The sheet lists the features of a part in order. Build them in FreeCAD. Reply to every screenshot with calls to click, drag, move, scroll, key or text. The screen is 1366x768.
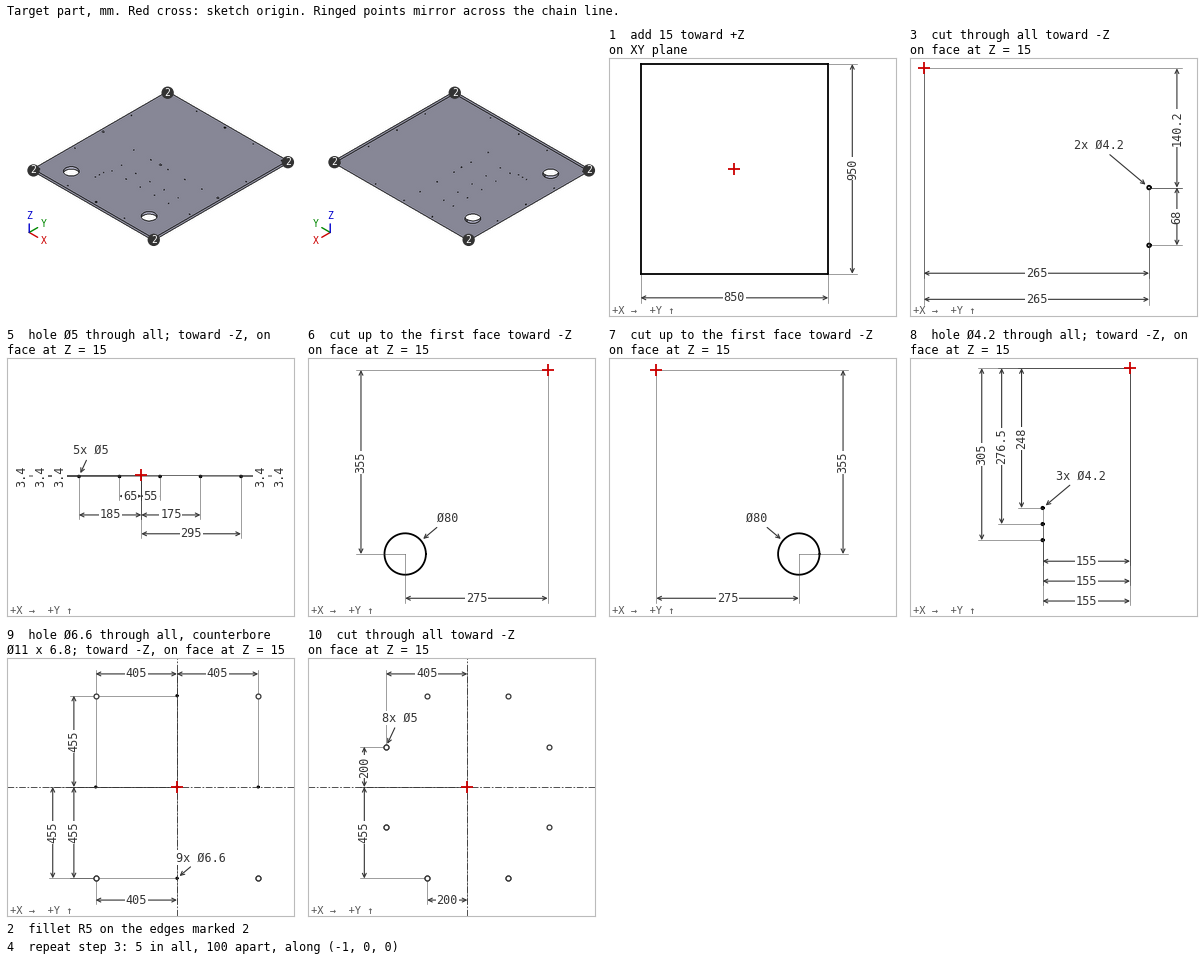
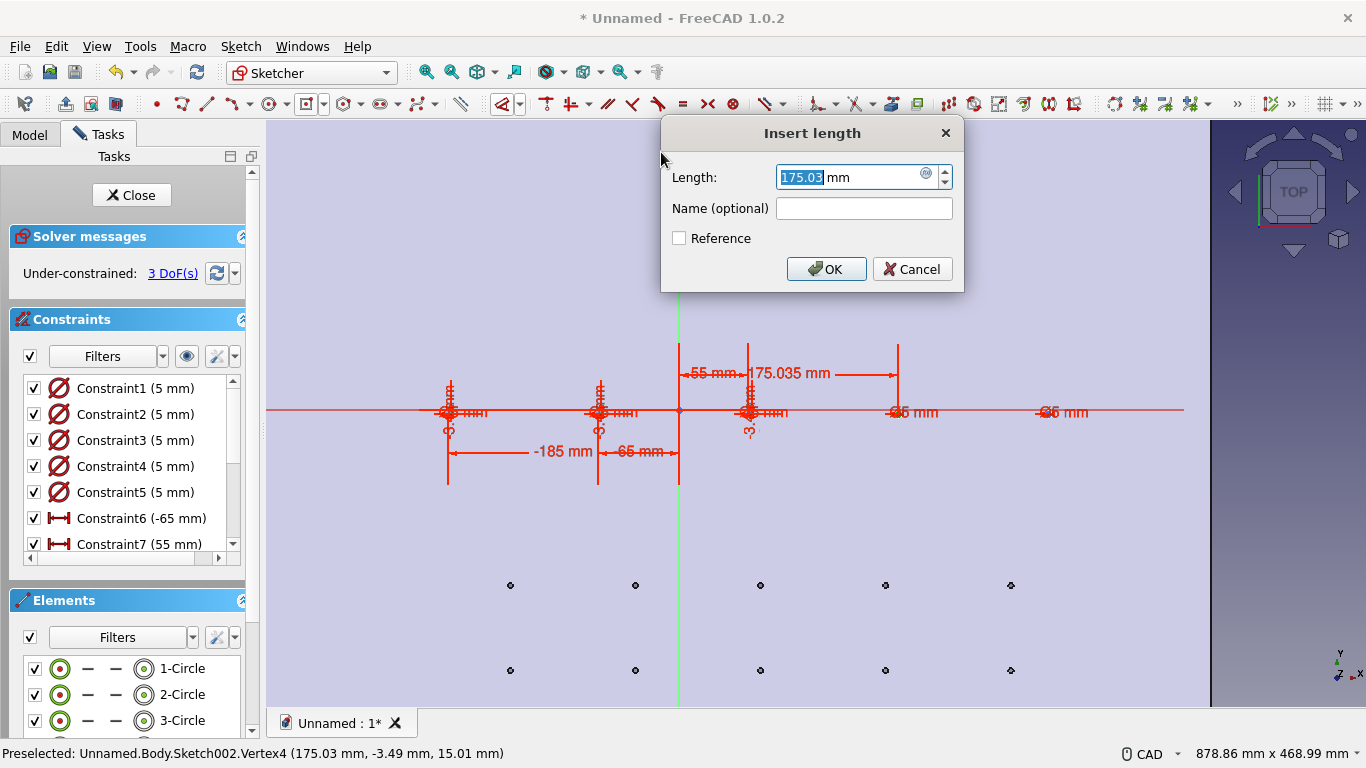
text(175)
key(Return)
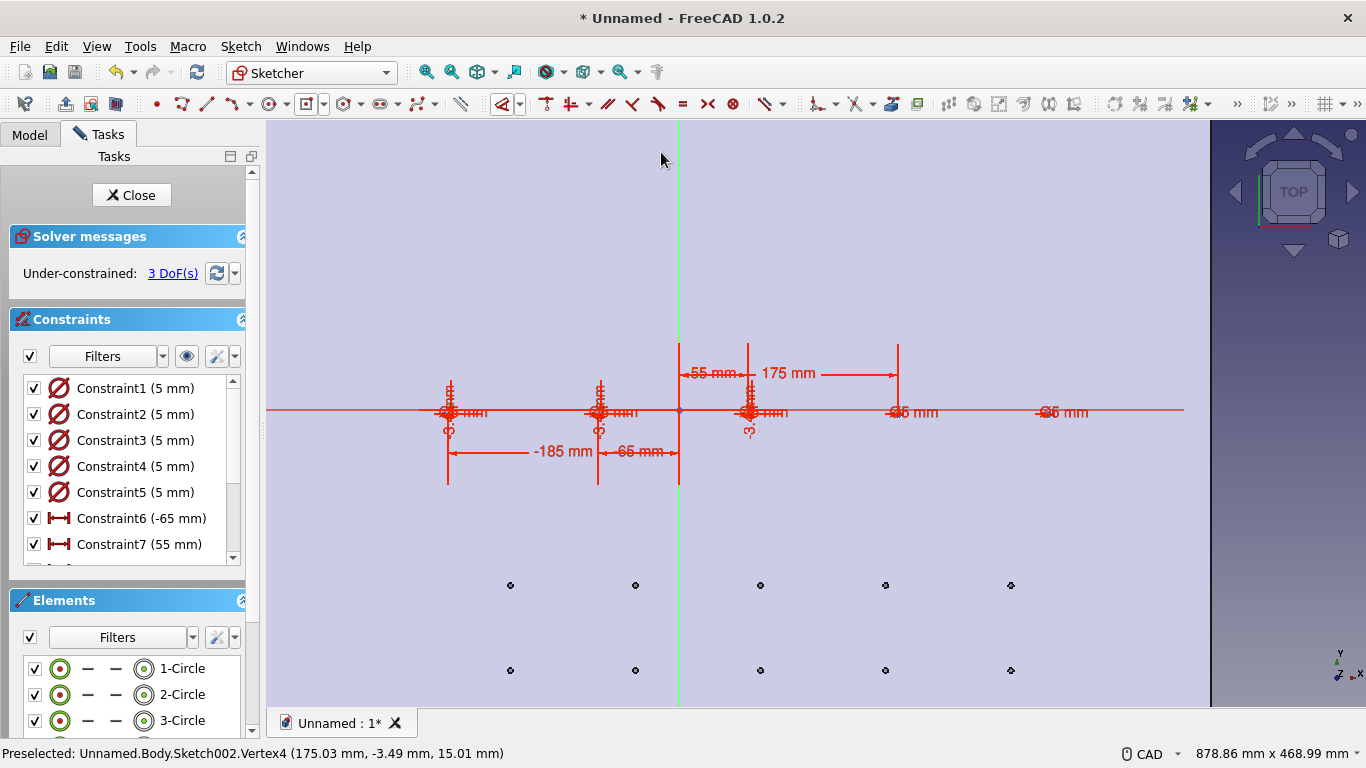
scroll(898, 414, up, 12)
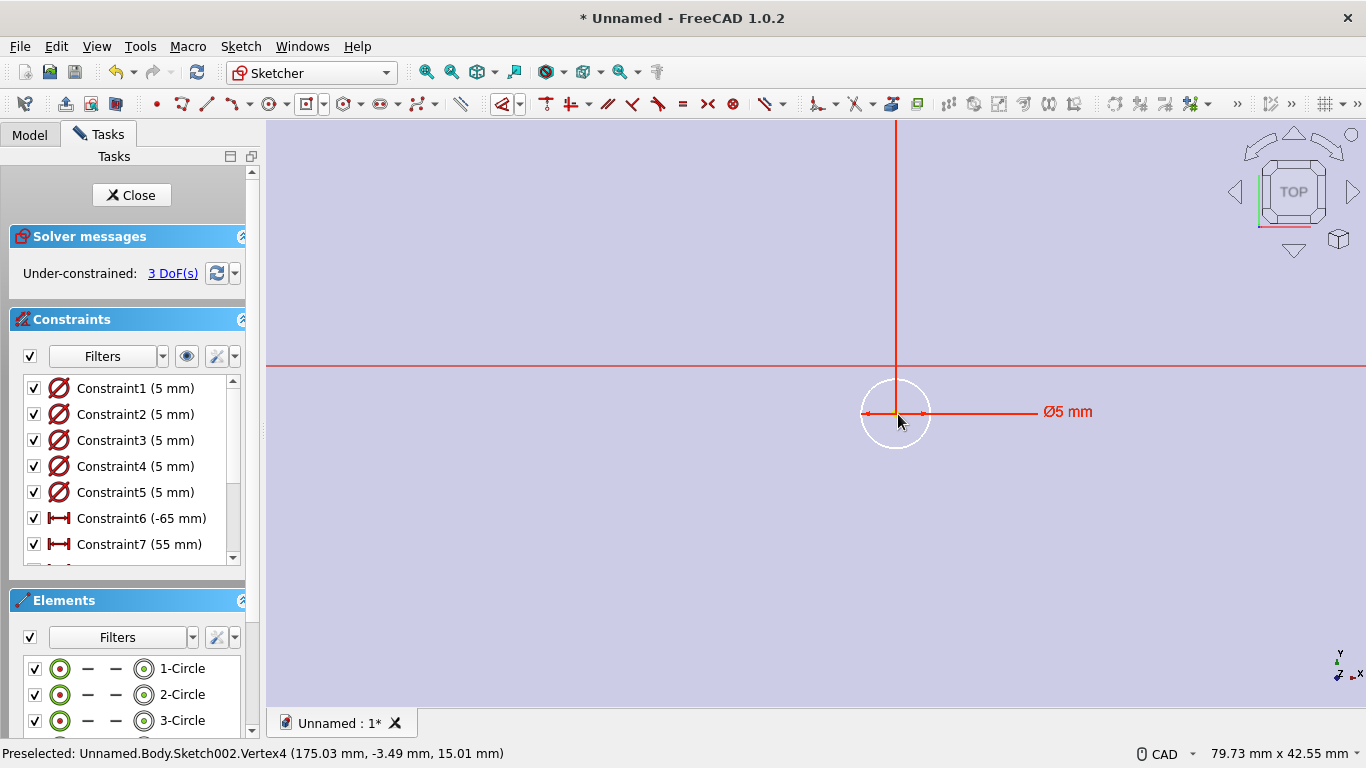
click(896, 414)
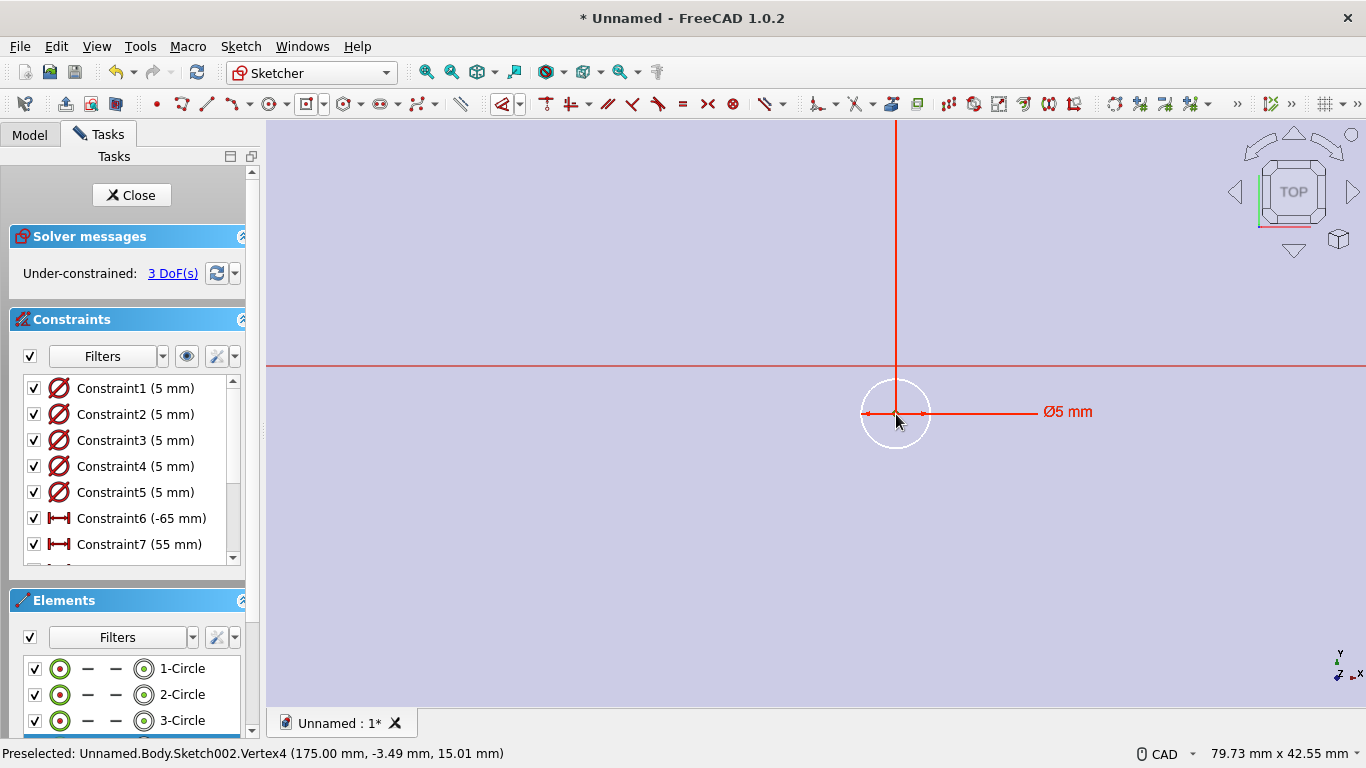
click(520, 104)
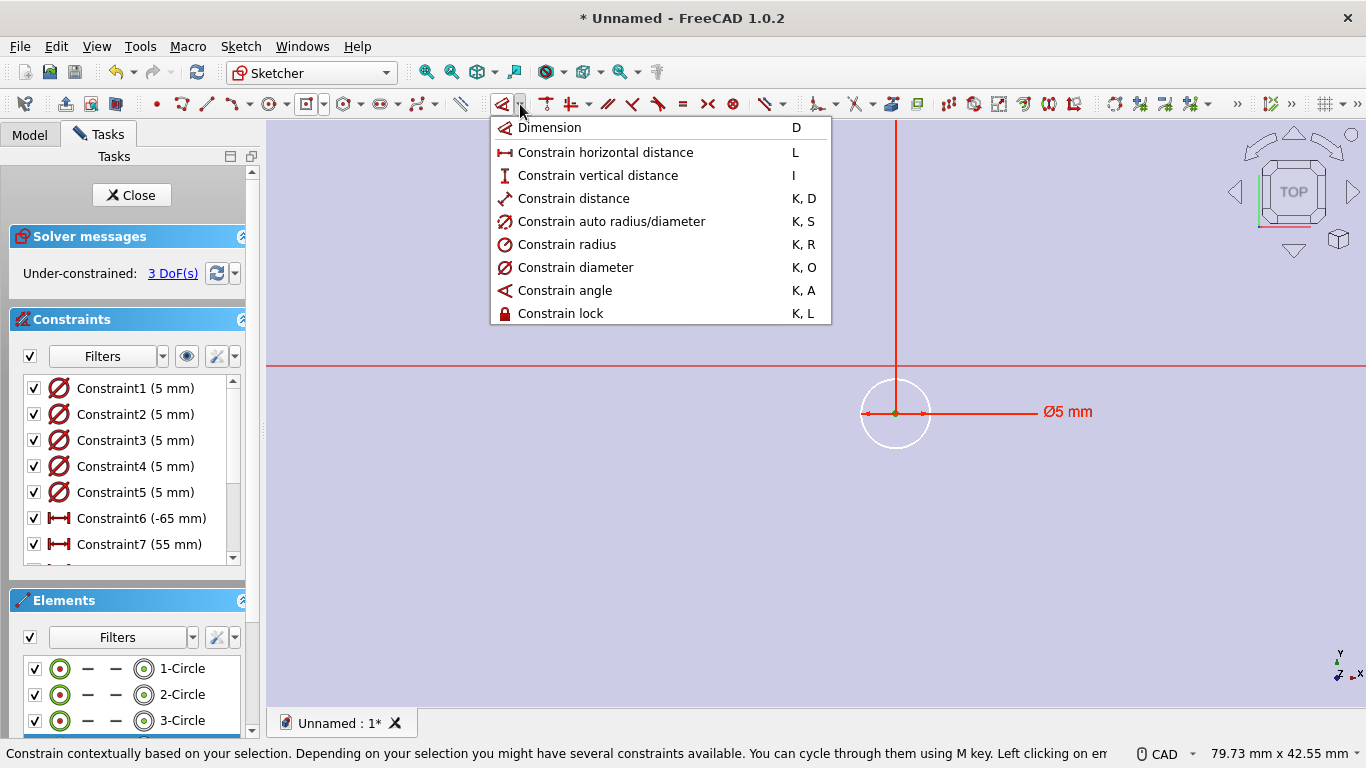
click(661, 176)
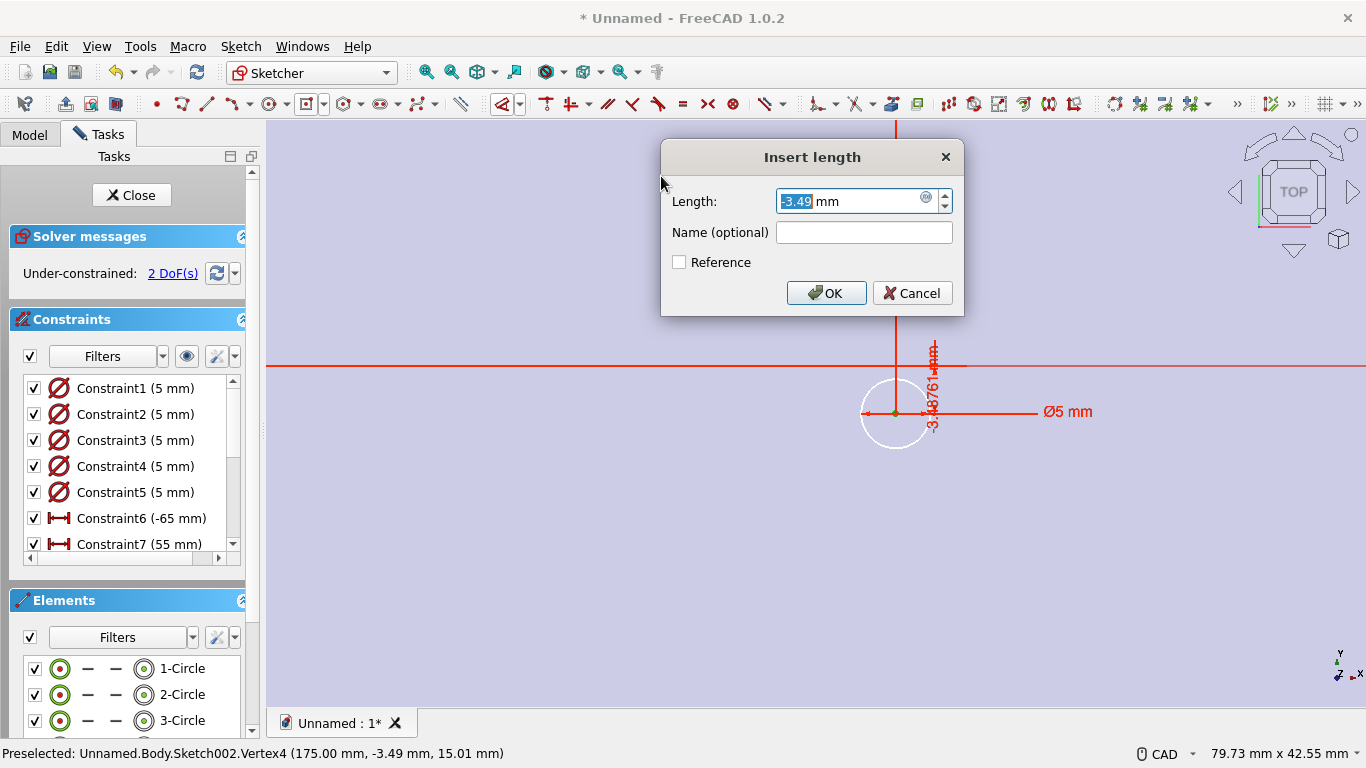
text(-3.4)
key(Return)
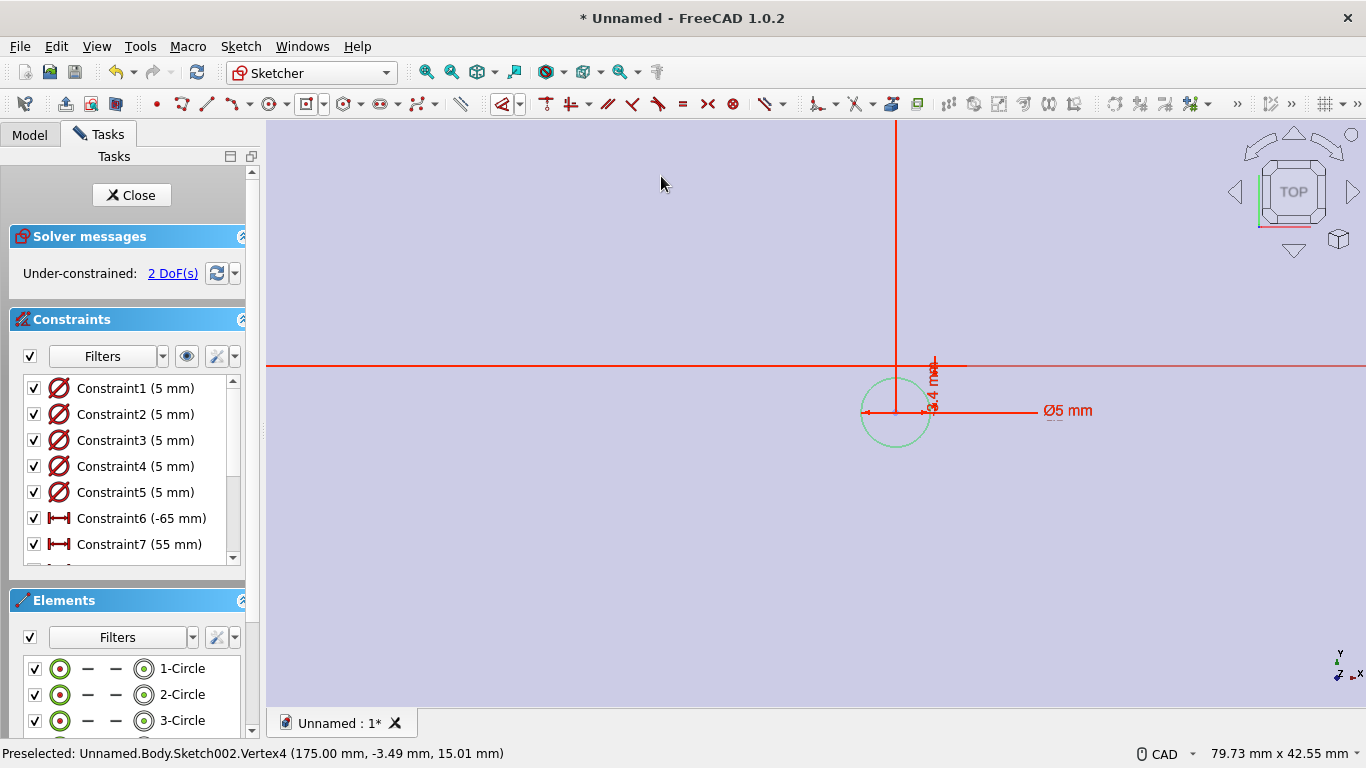
scroll(898, 414, down, 12)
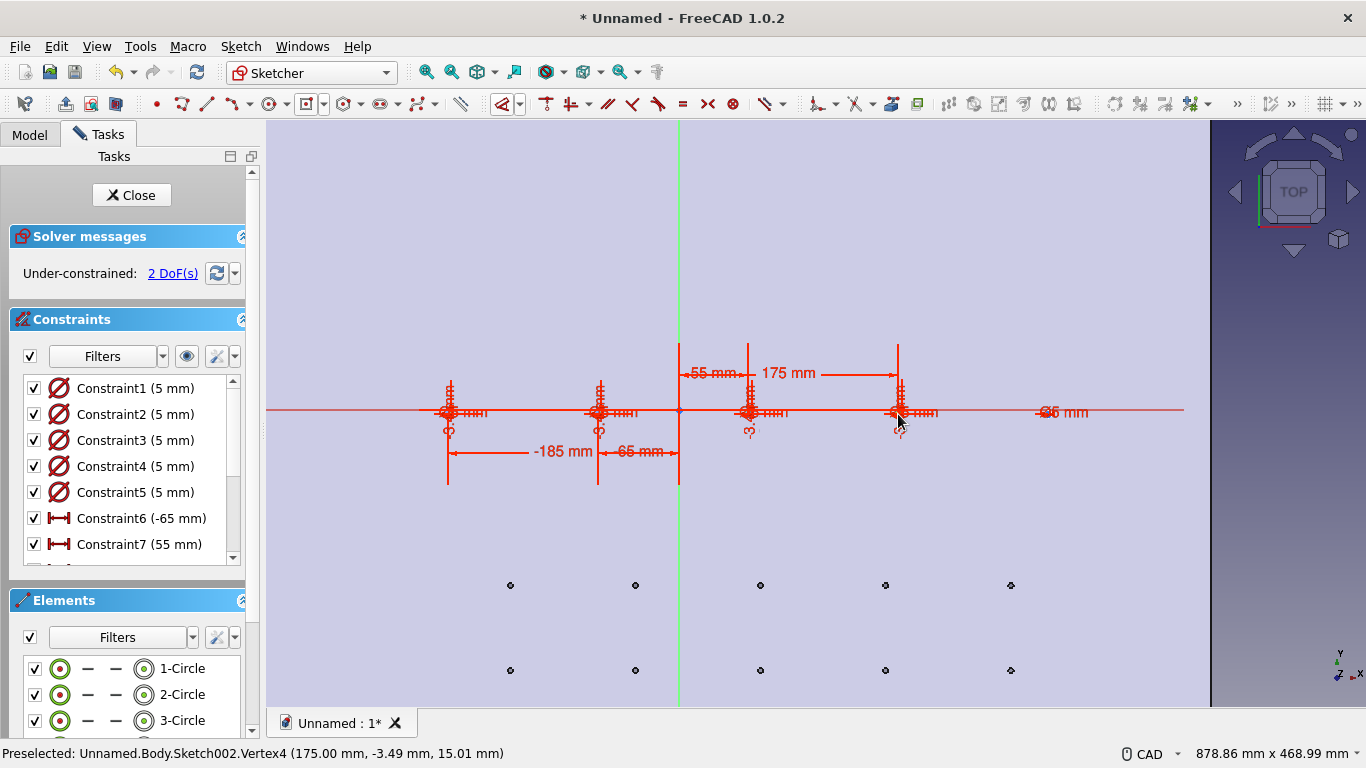
click(1049, 414)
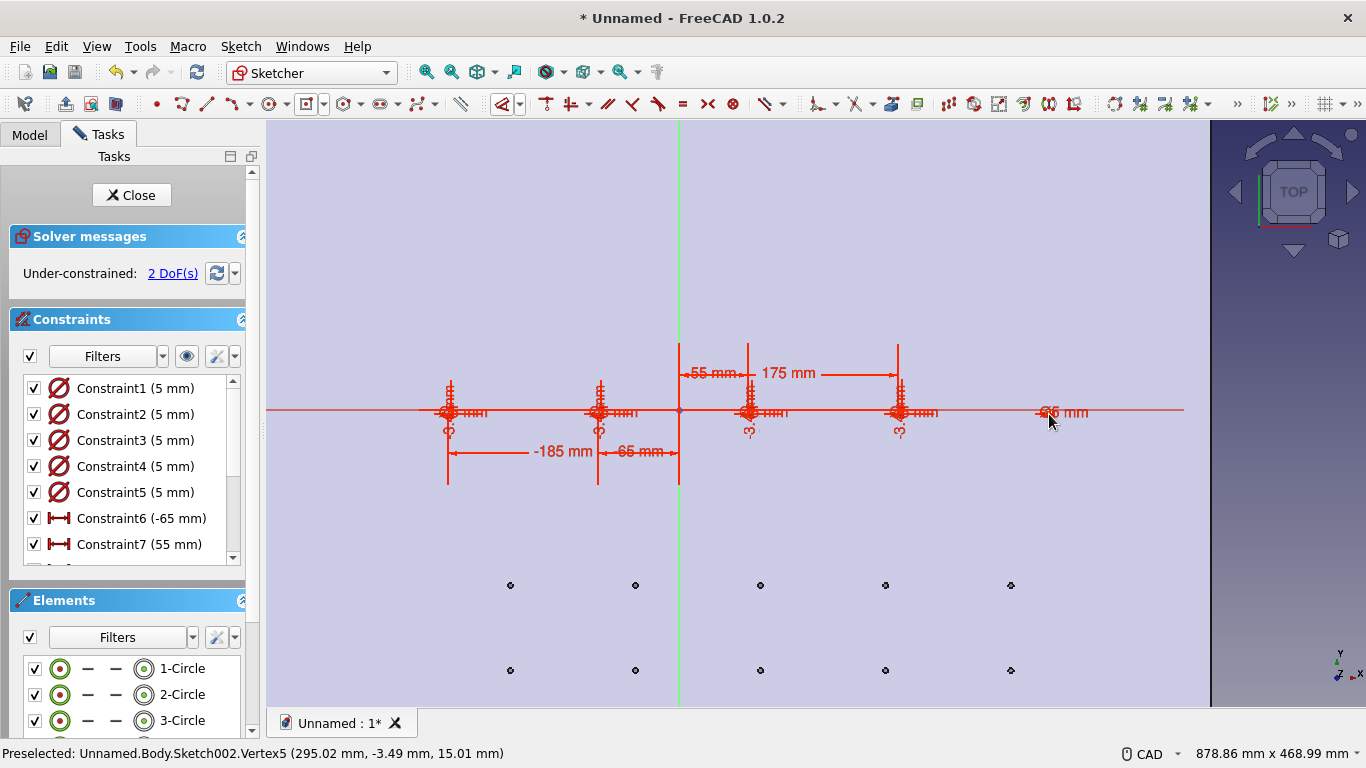
key(l)